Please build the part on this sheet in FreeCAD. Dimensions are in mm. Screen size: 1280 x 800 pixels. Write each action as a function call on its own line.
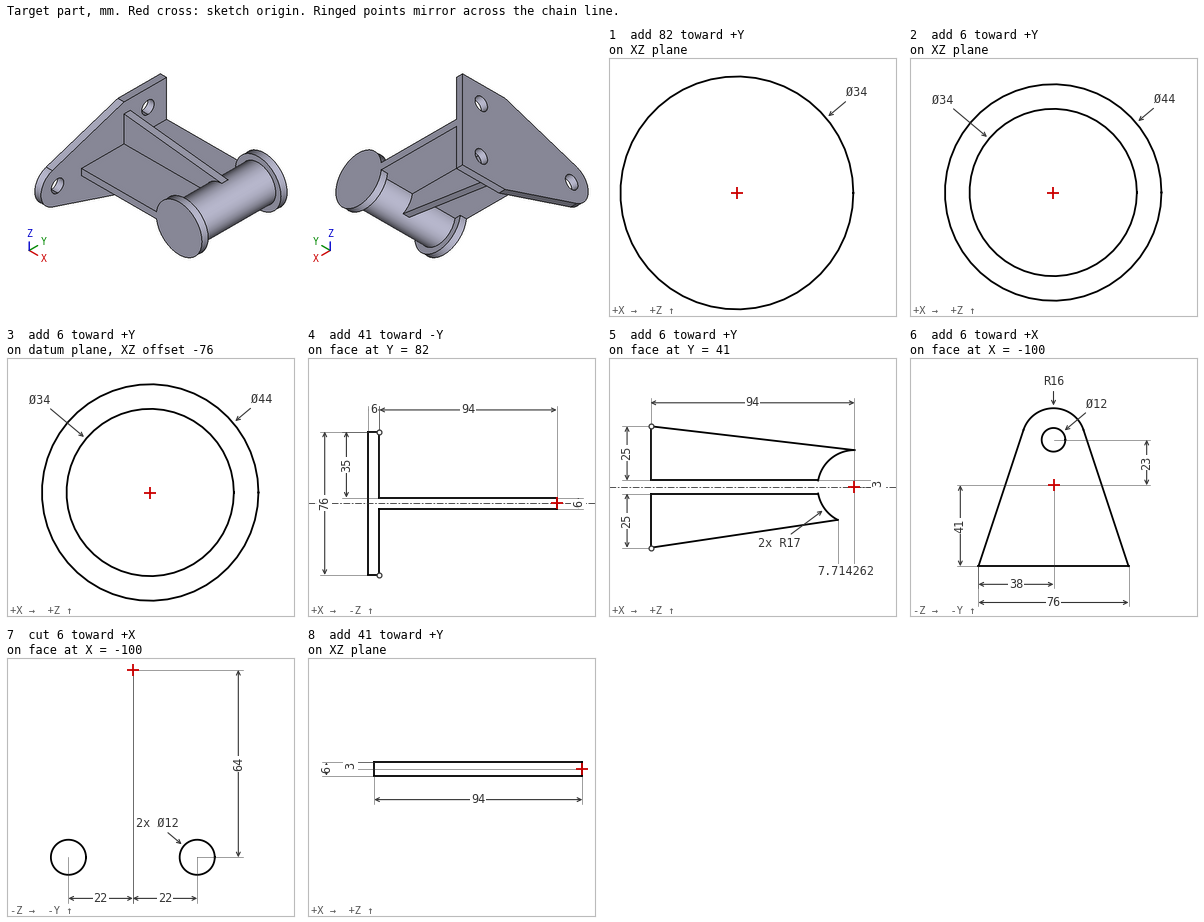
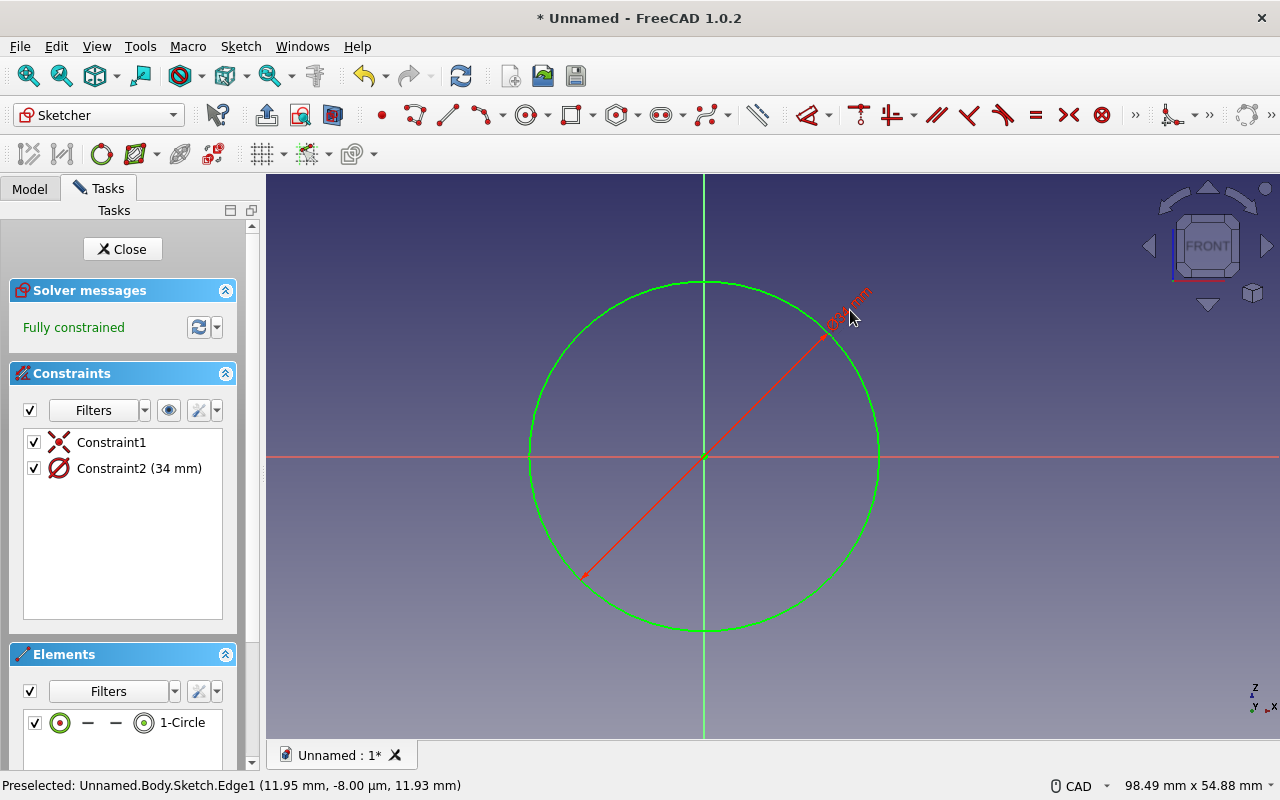
click(123, 249)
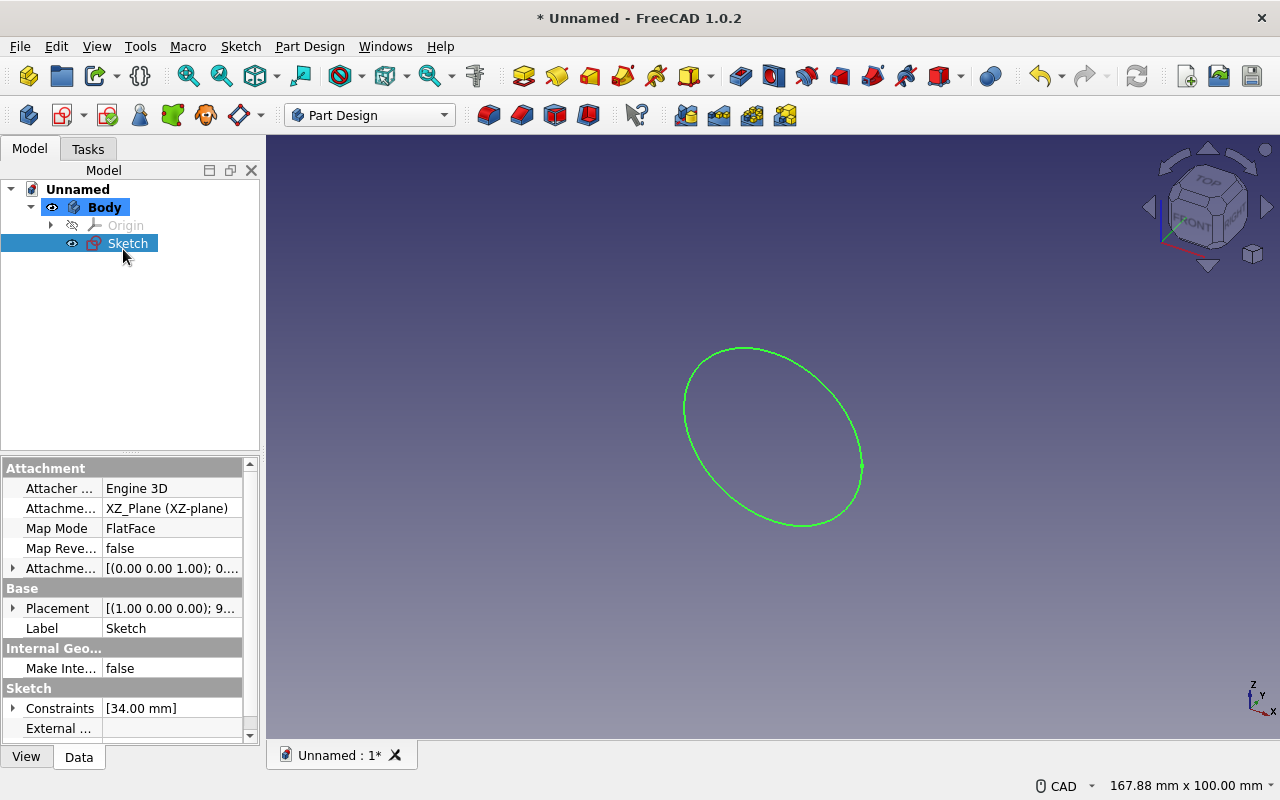
click(524, 76)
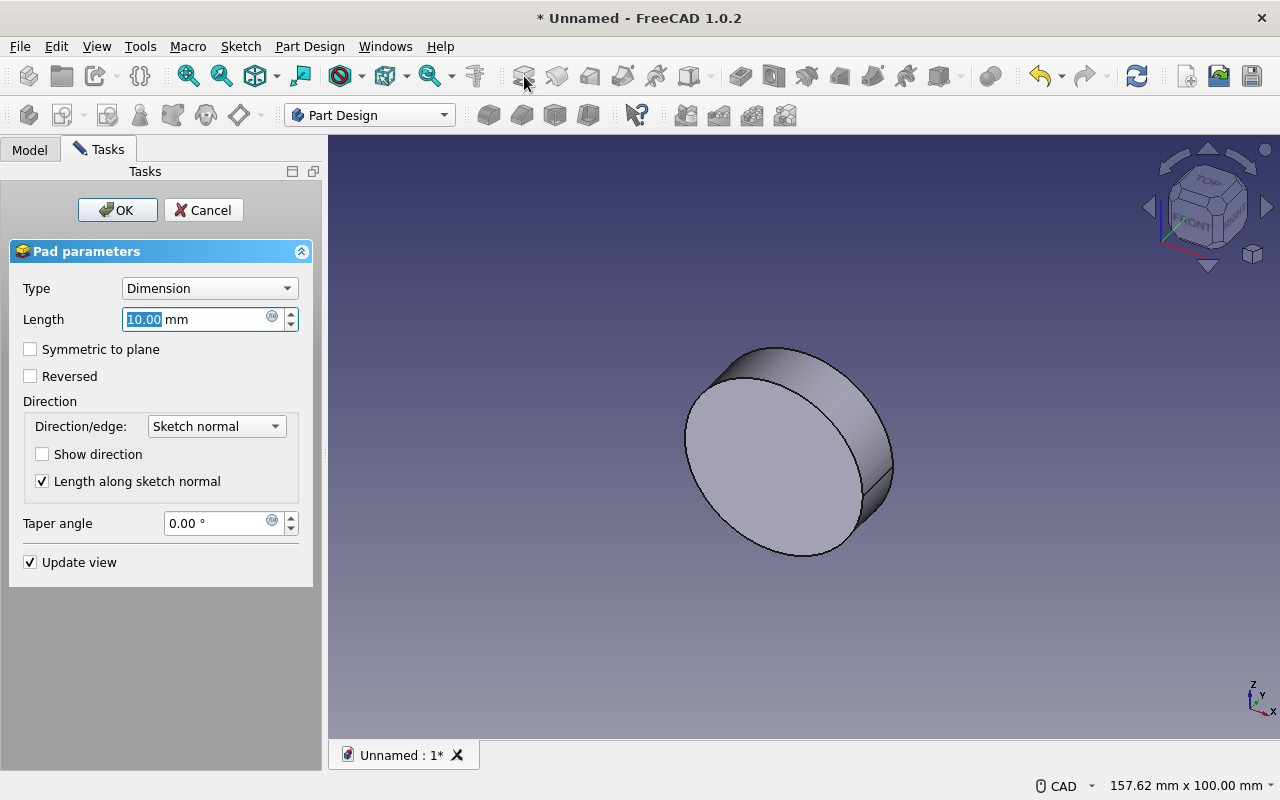
text(82)
key(Tab)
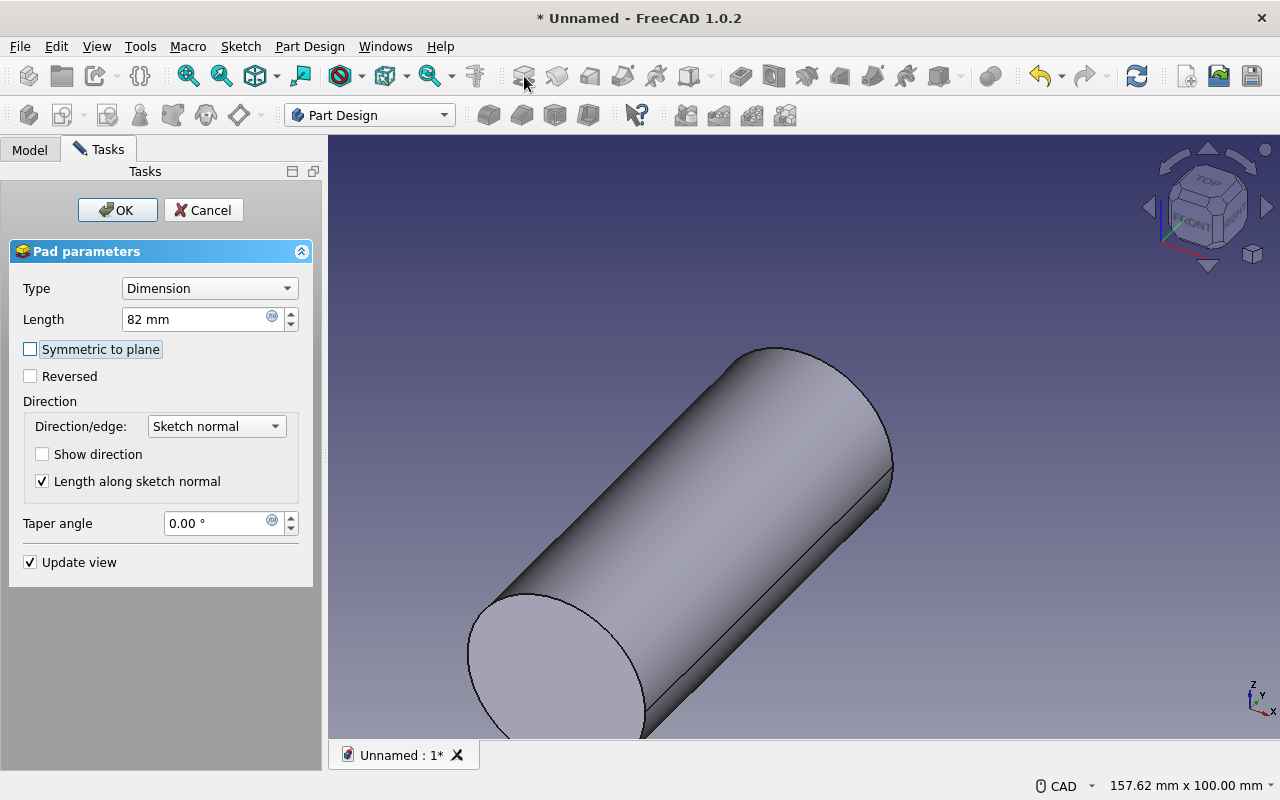
click(31, 376)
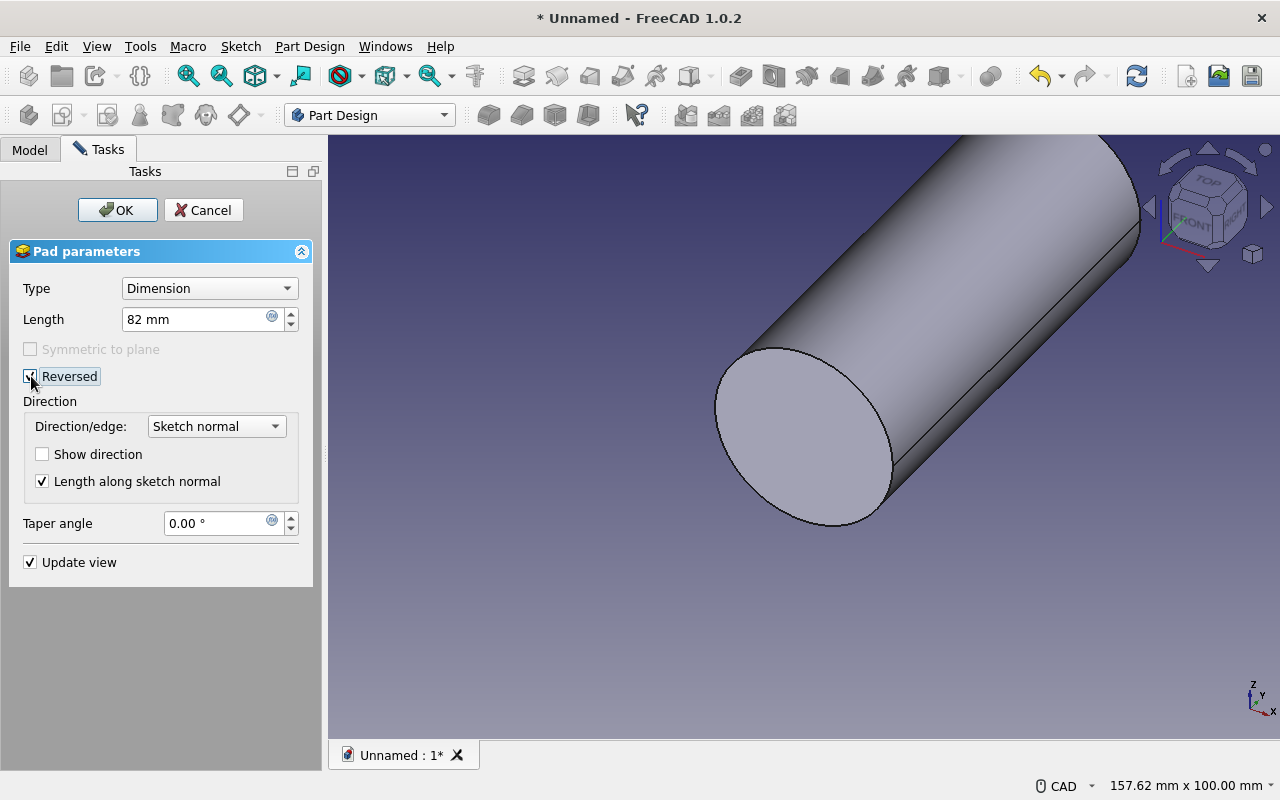
click(118, 210)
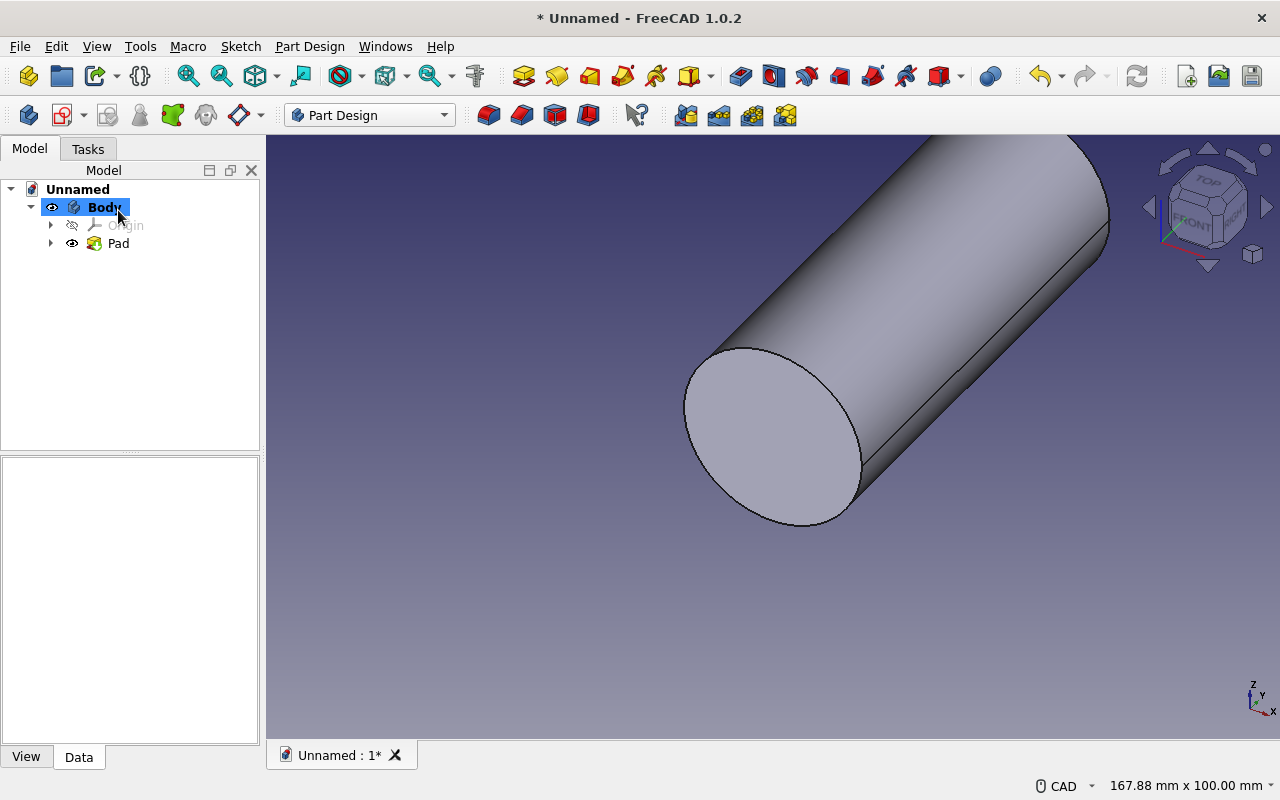
click(189, 76)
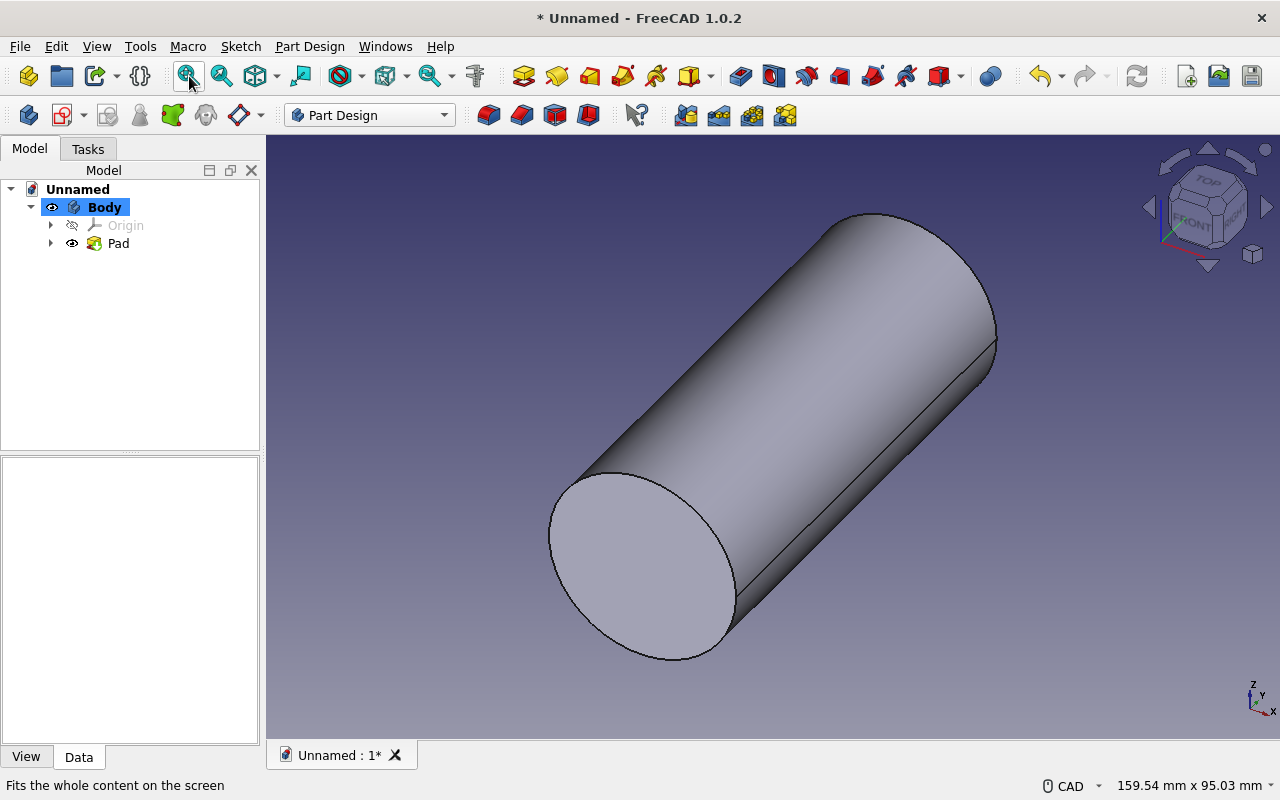
click(62, 116)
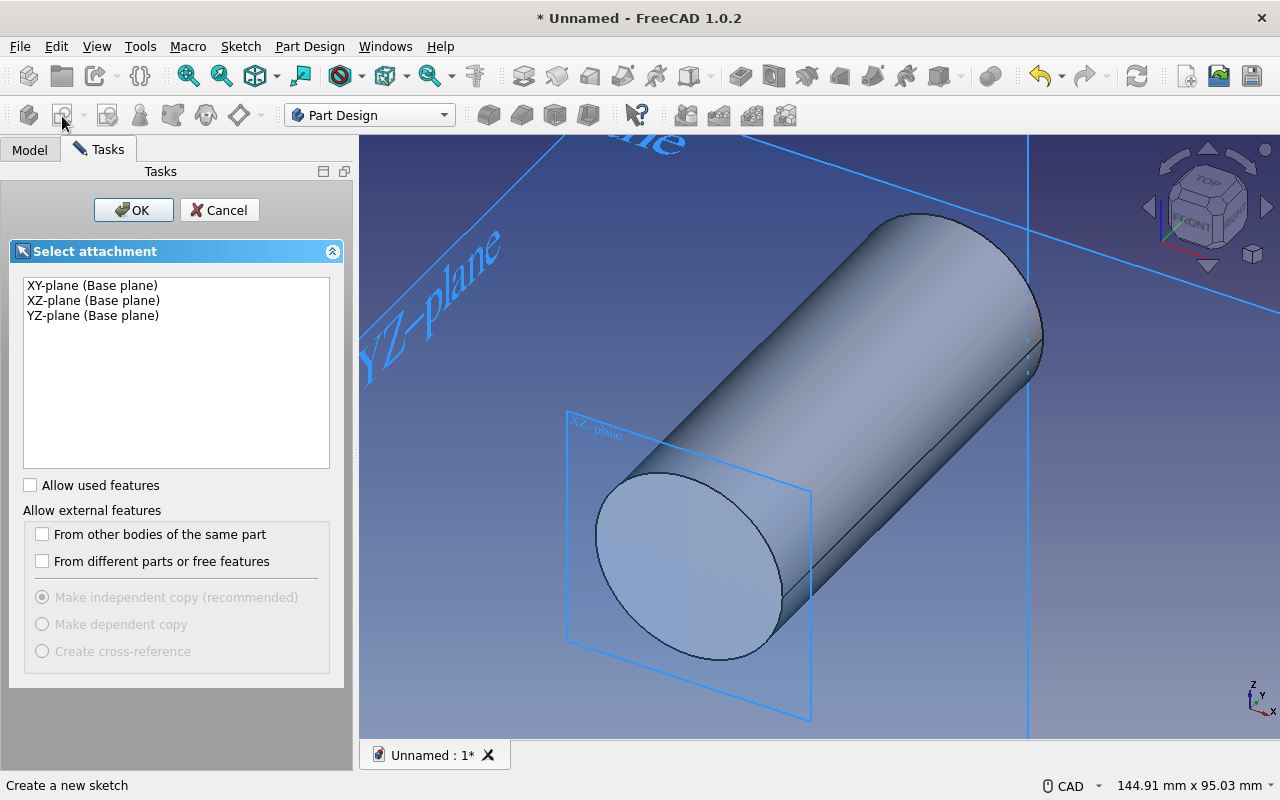
click(84, 300)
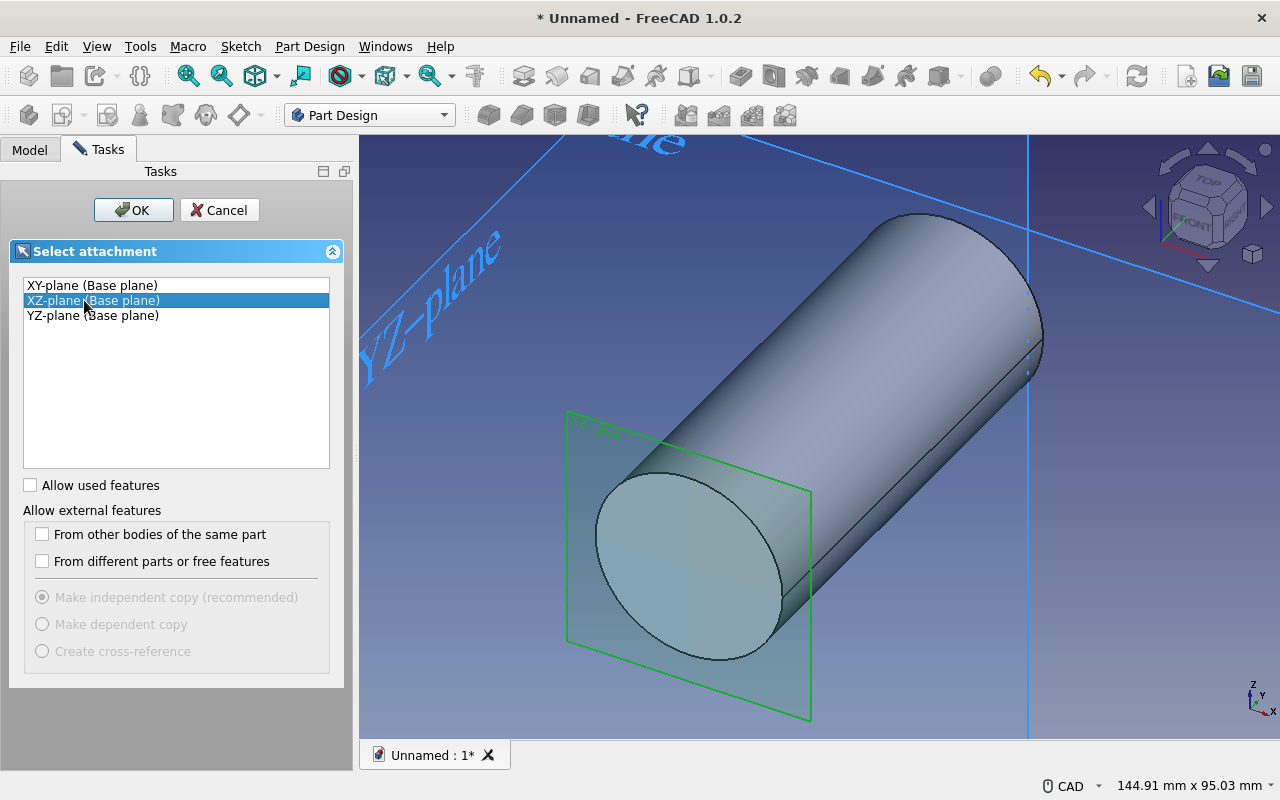
click(134, 210)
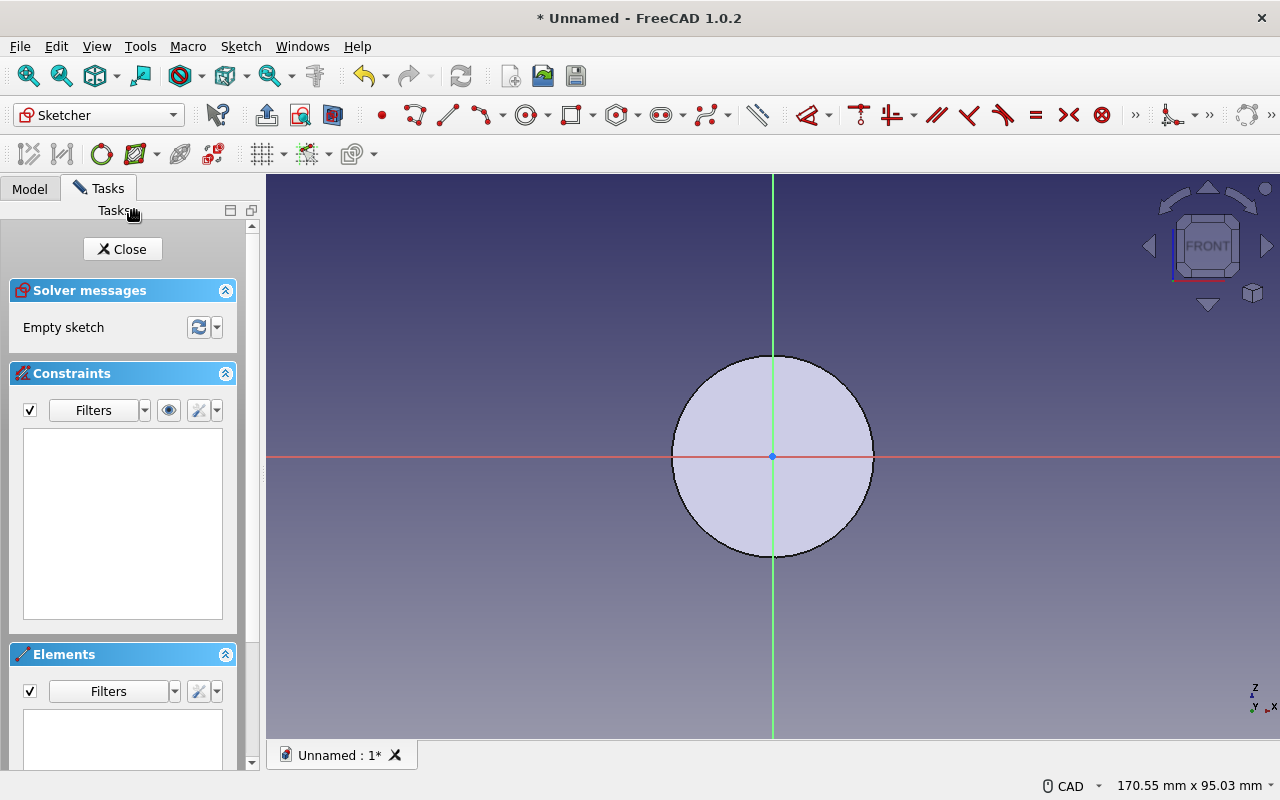
scroll(912, 457, up, 2)